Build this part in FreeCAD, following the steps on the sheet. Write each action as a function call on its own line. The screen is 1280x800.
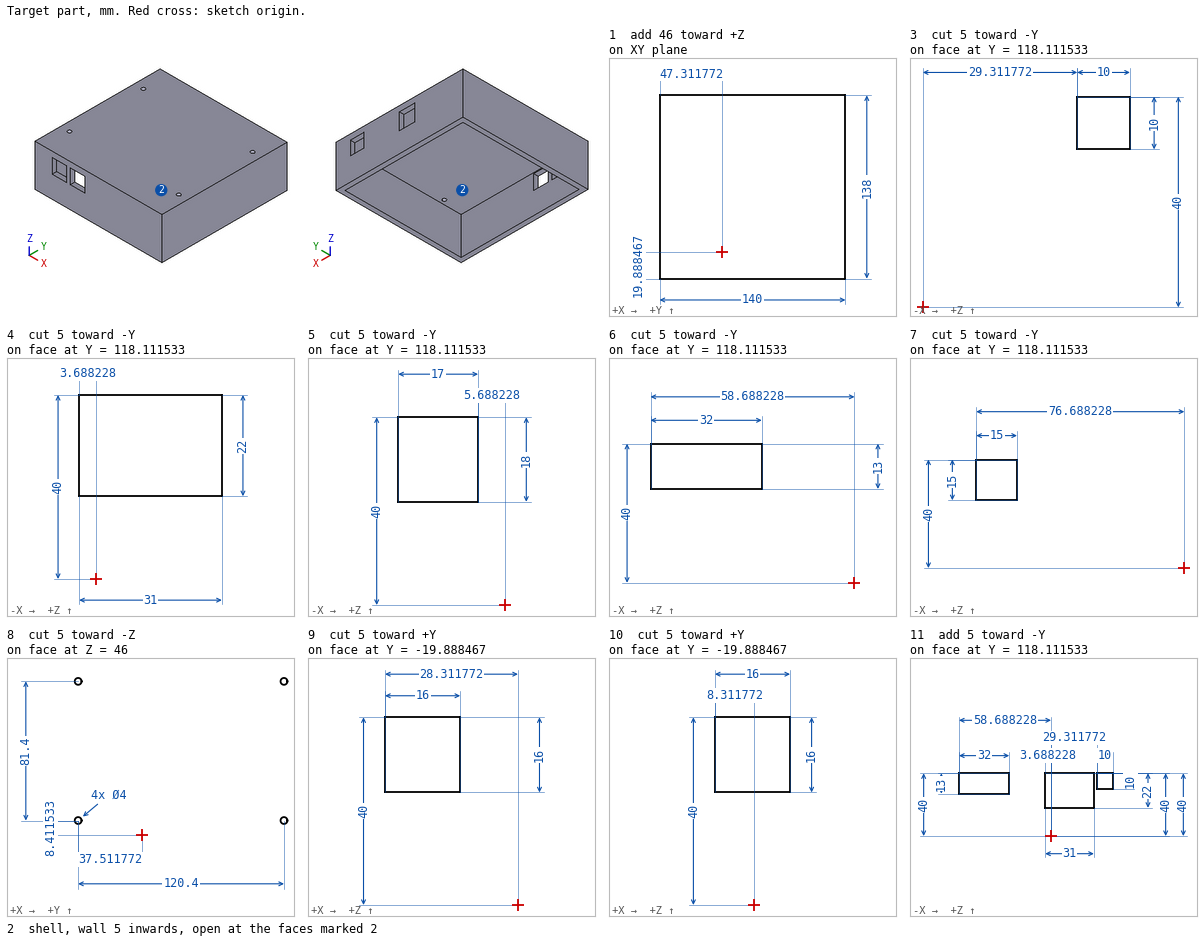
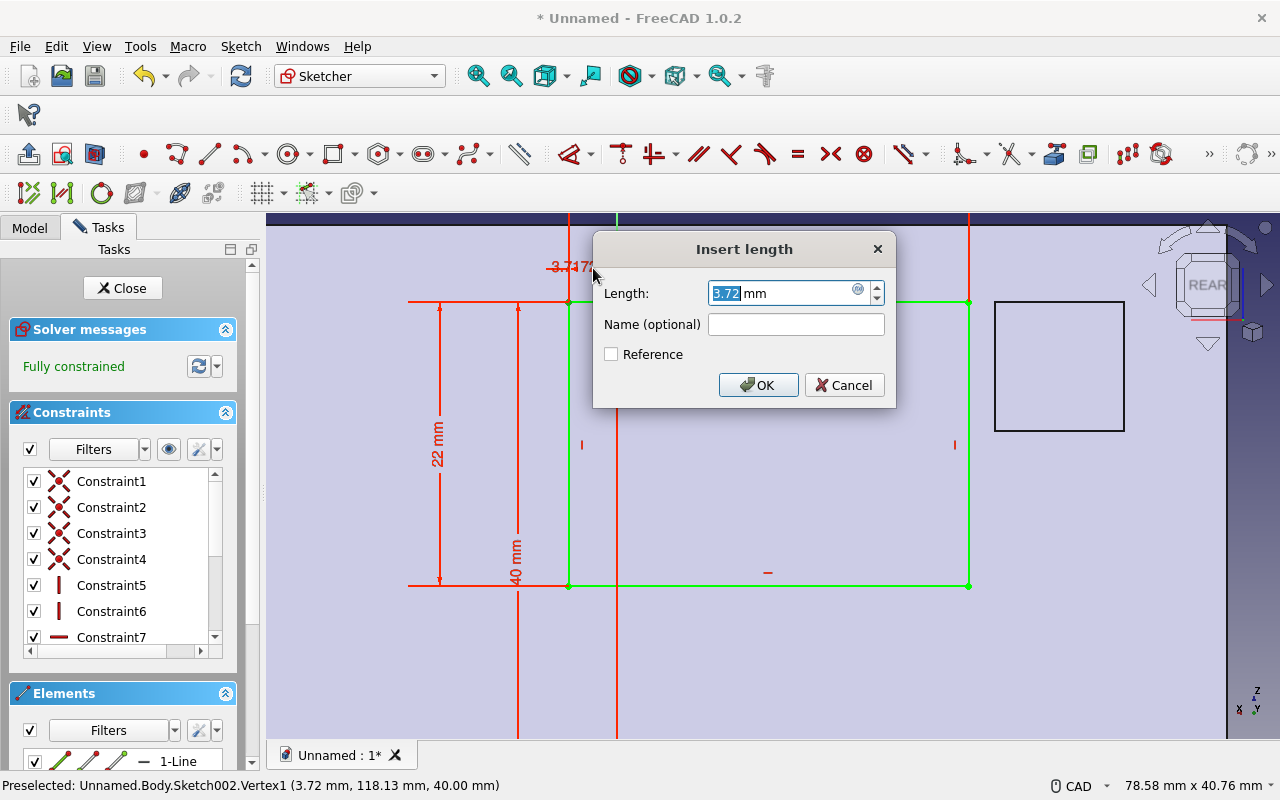
text(3.688228)
key(Return)
key(Escape)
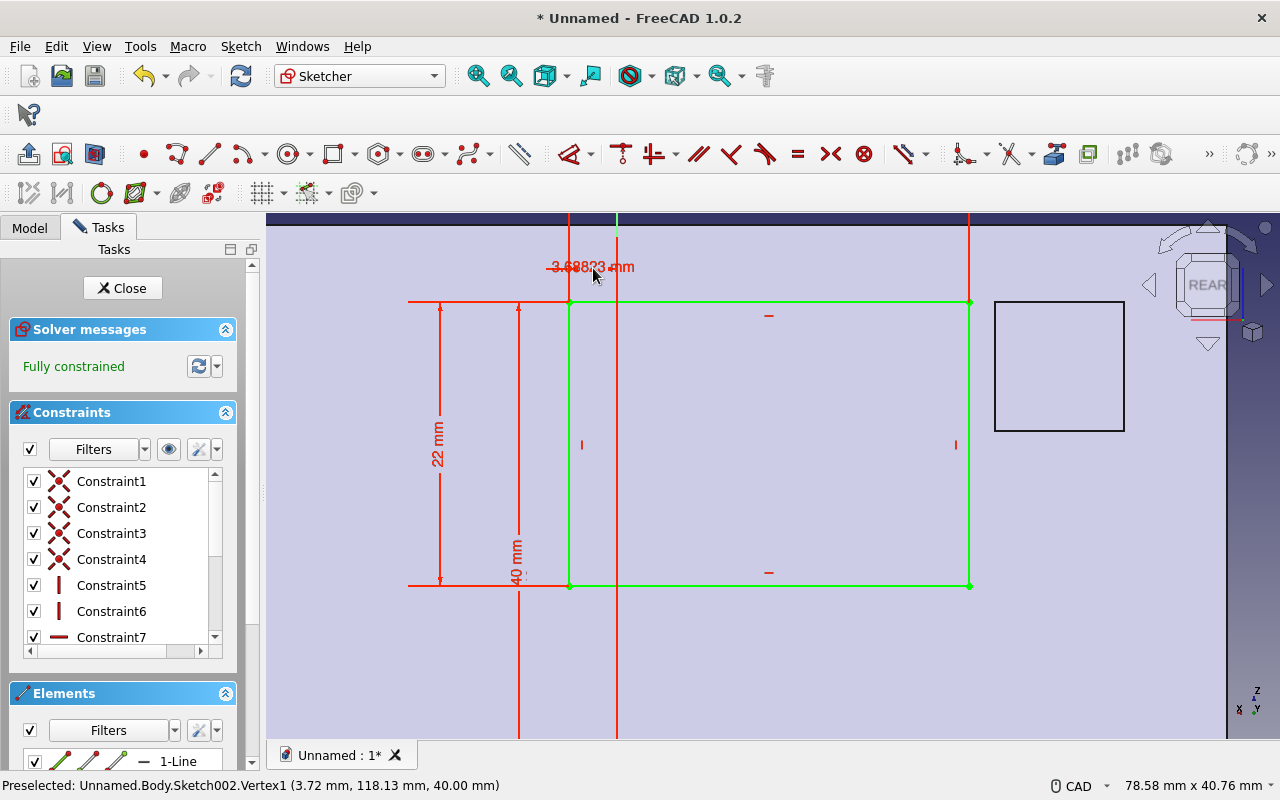
click(123, 288)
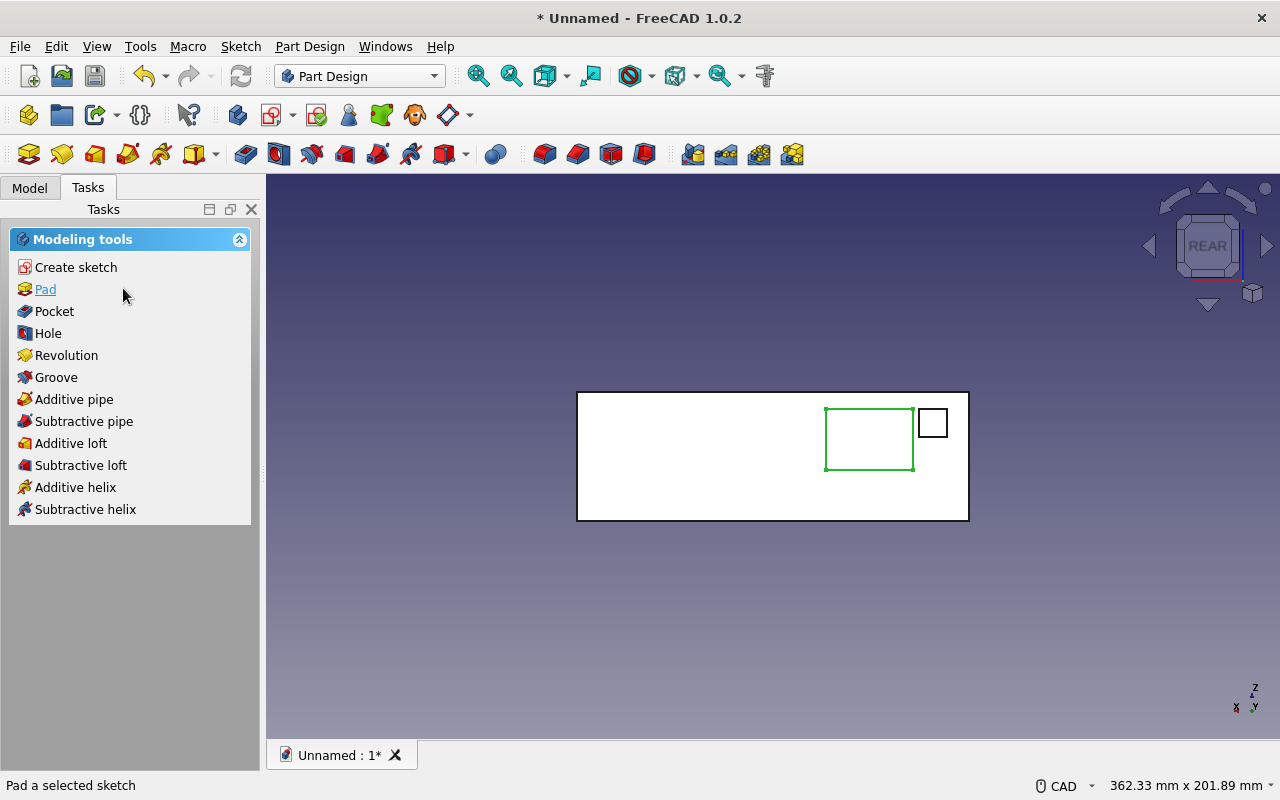
click(246, 154)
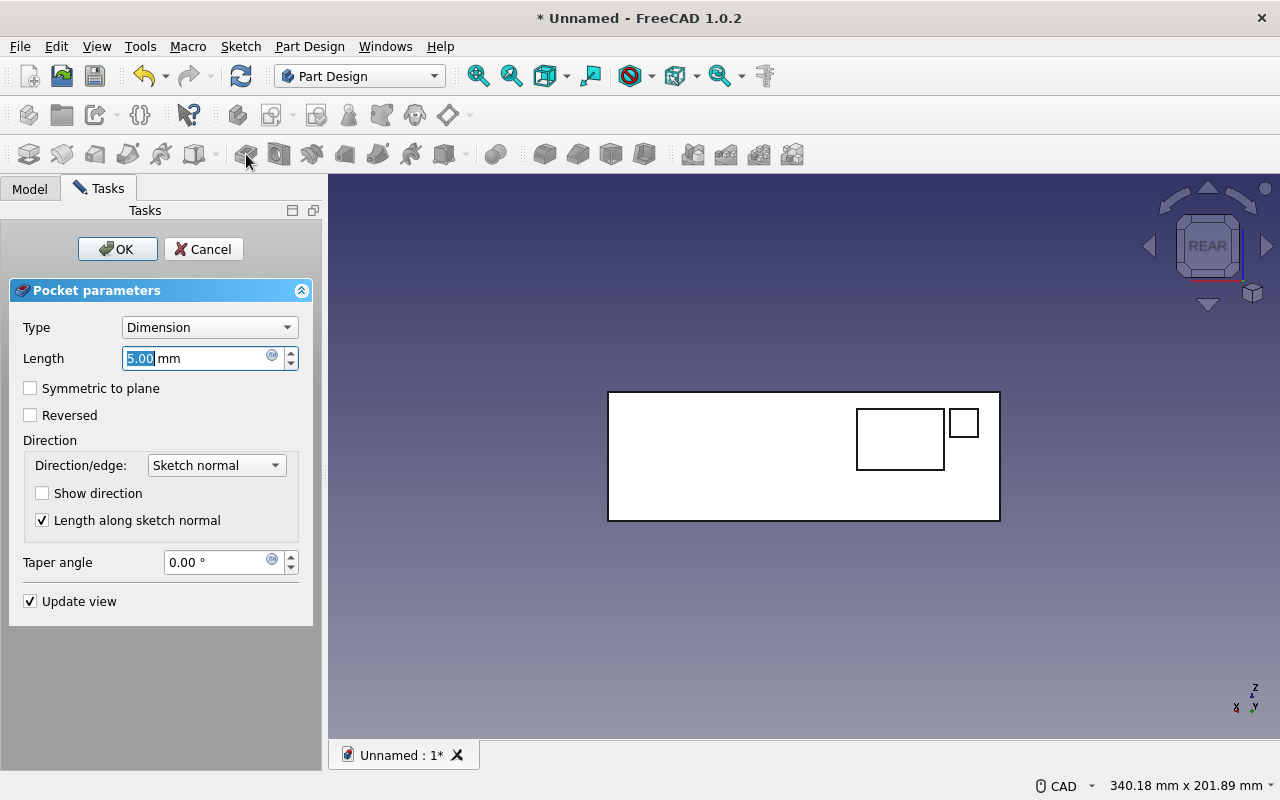
text(5)
key(Tab)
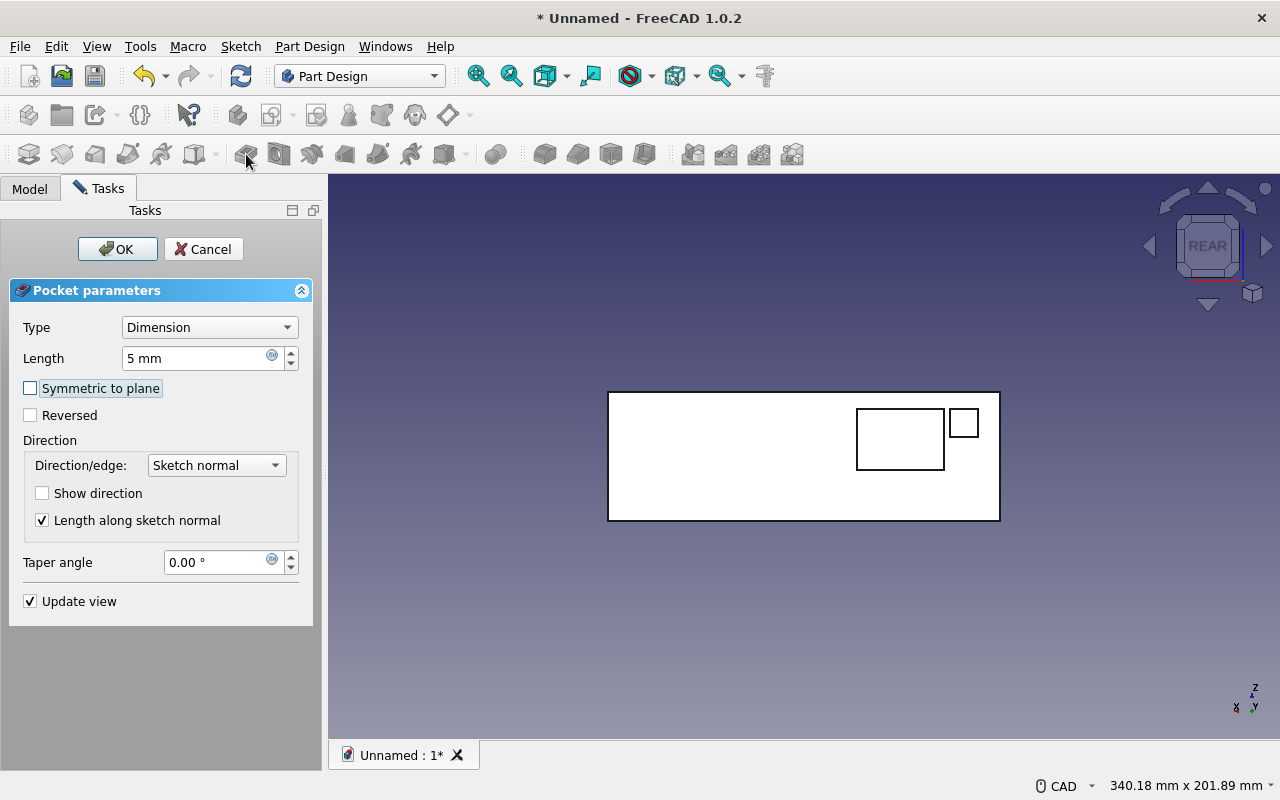
click(118, 249)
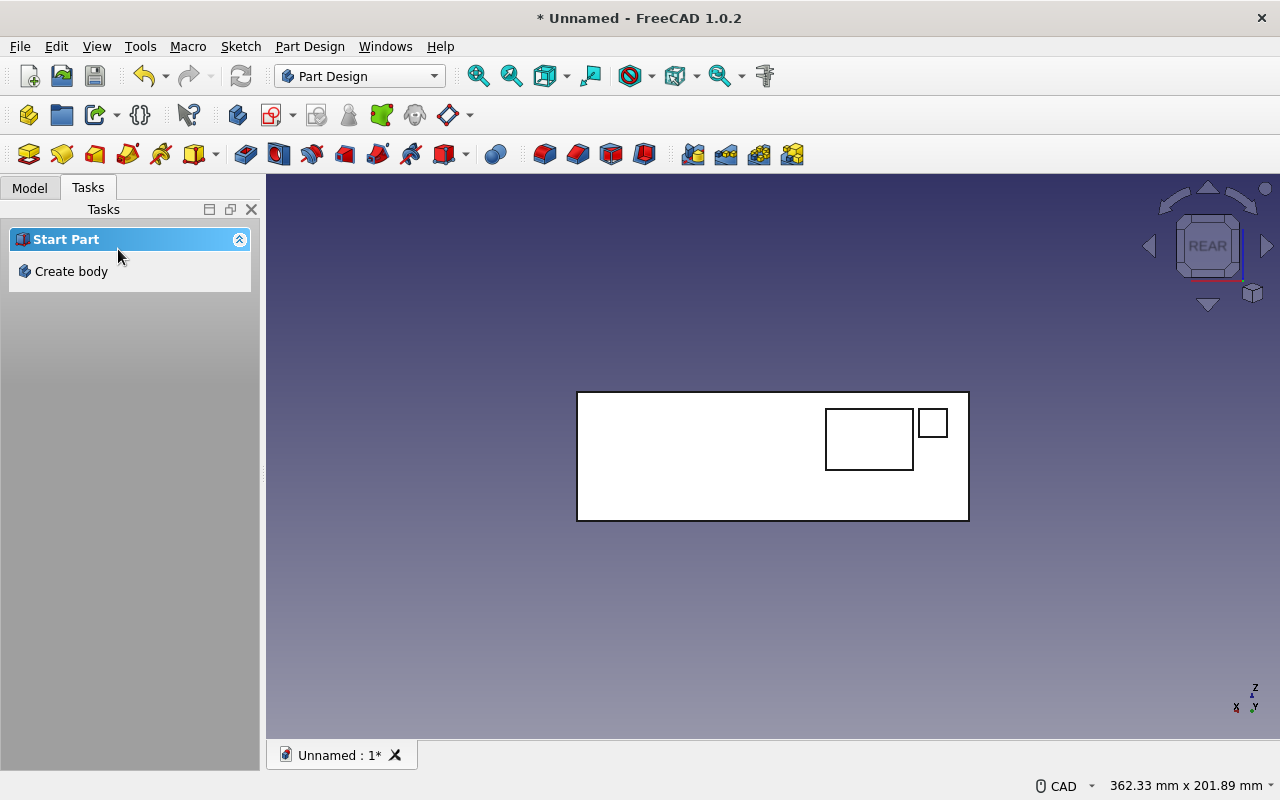
click(479, 76)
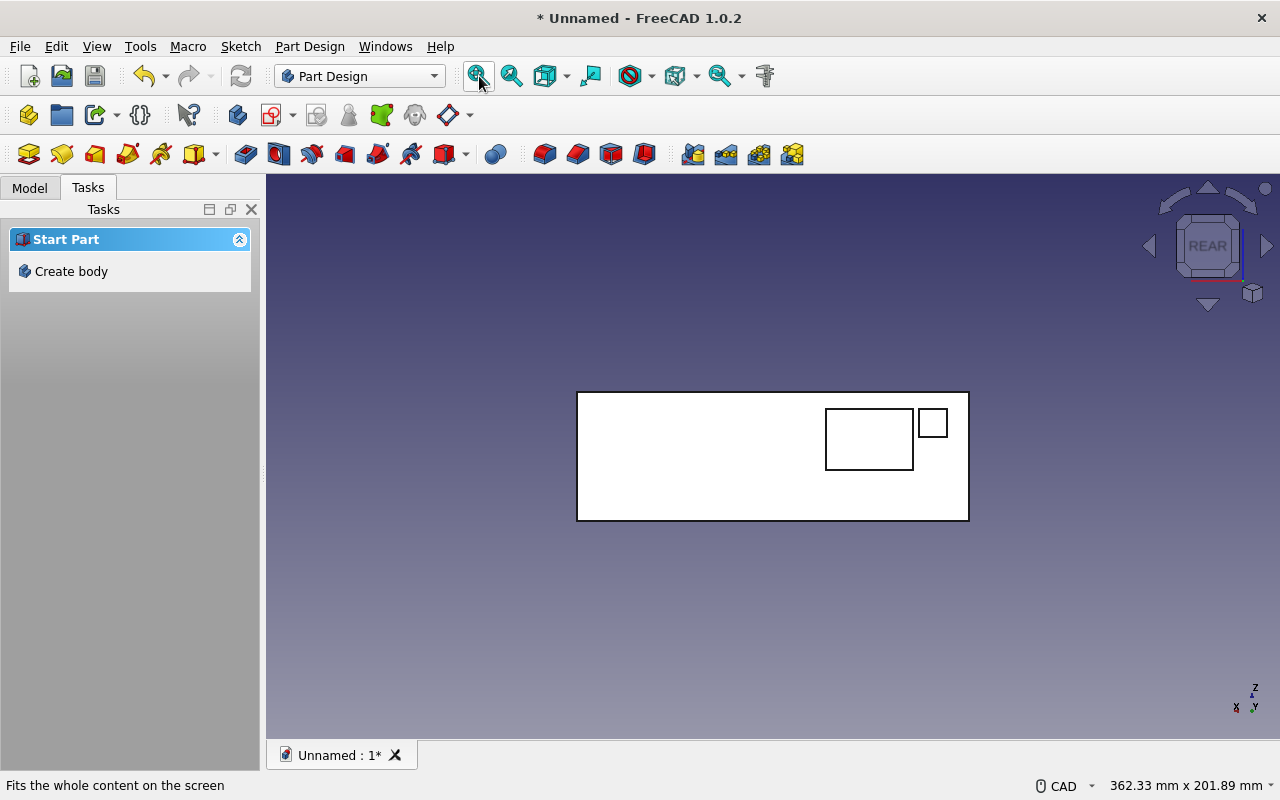
click(661, 455)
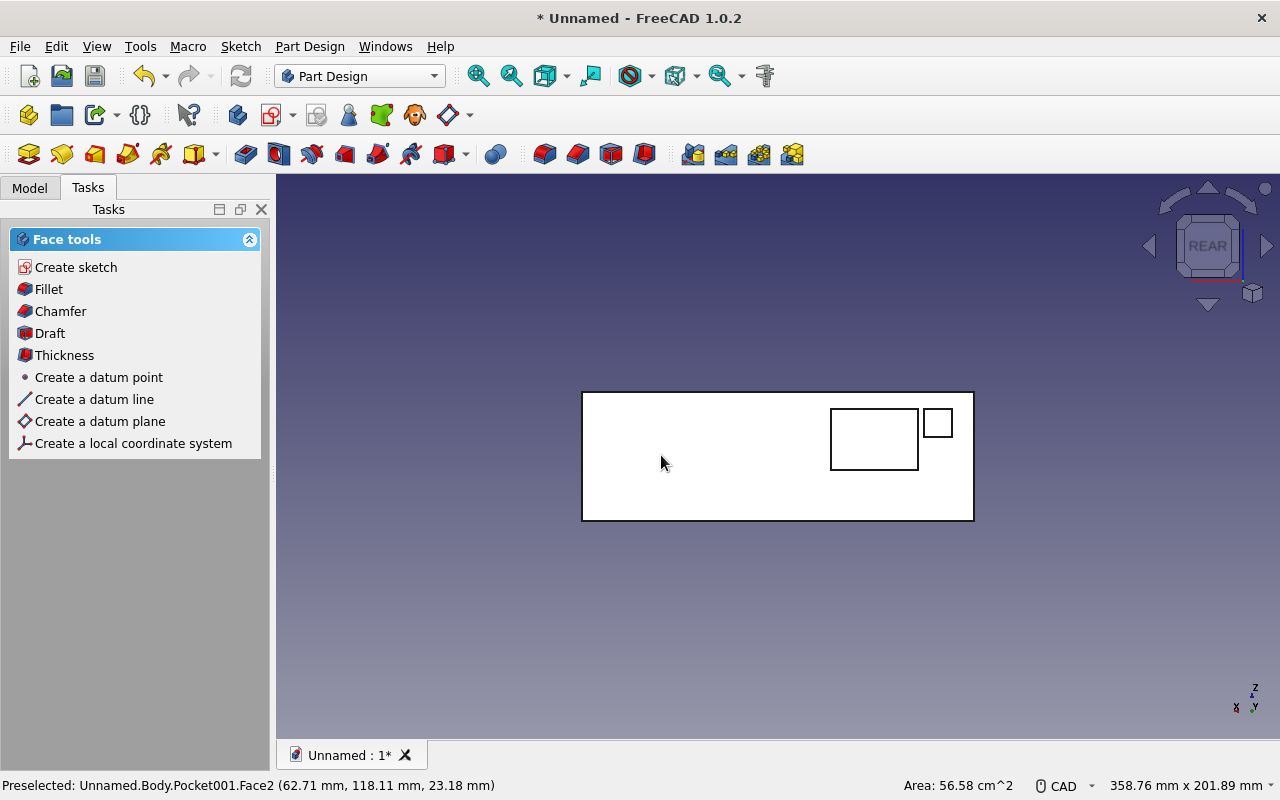
click(270, 116)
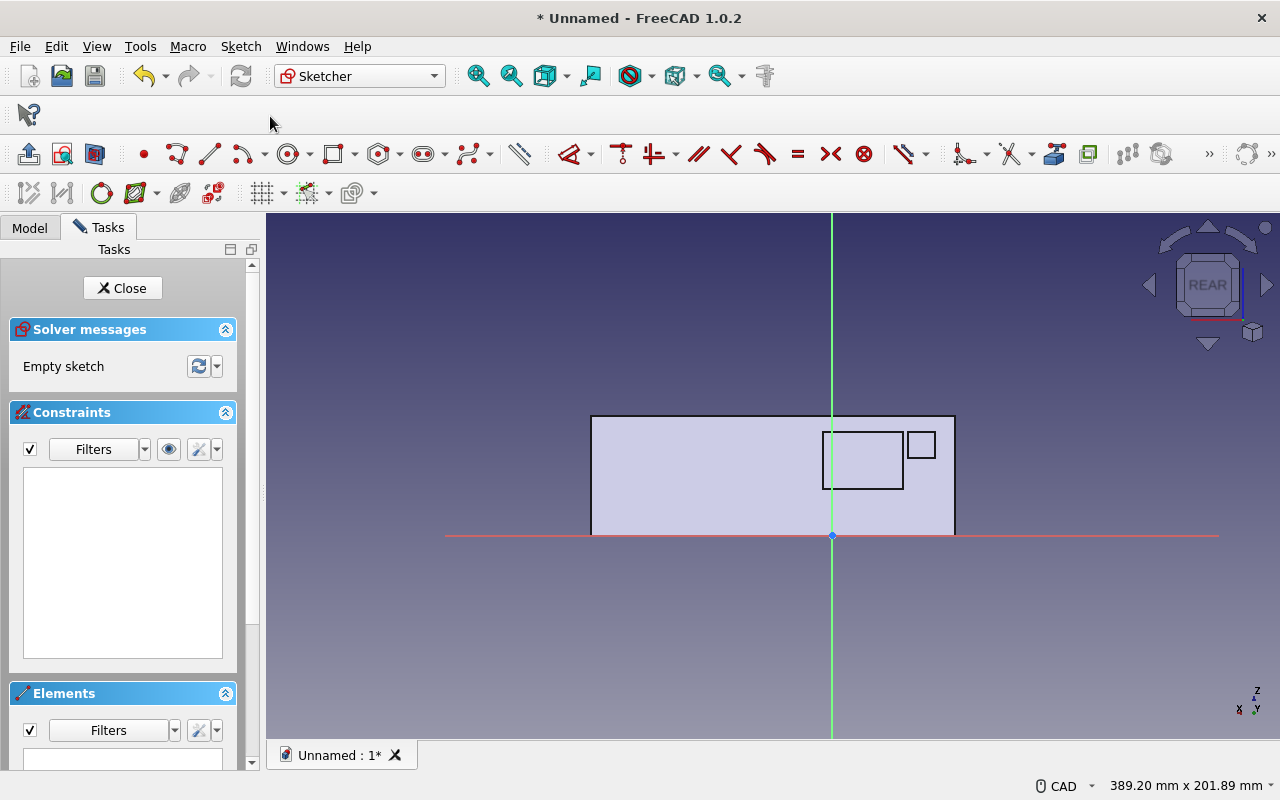
scroll(845, 487, up, 6)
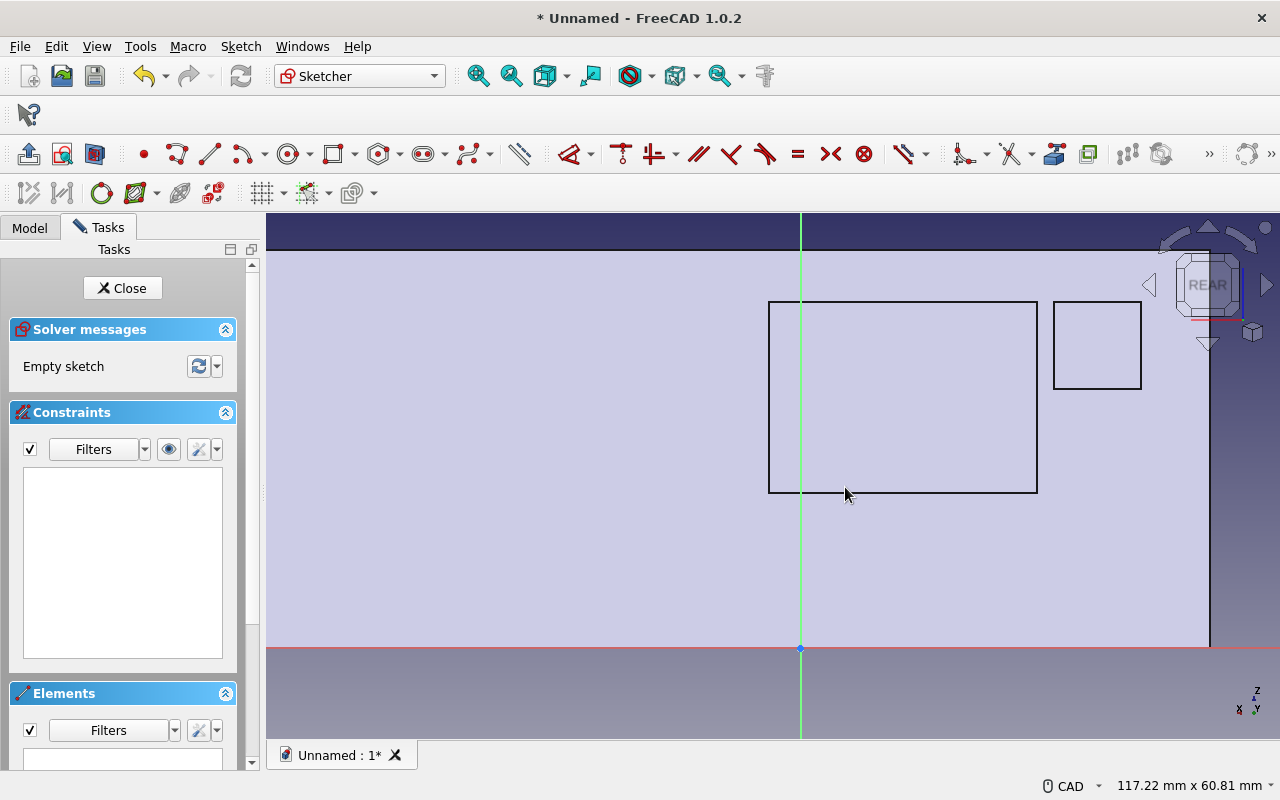
click(332, 154)